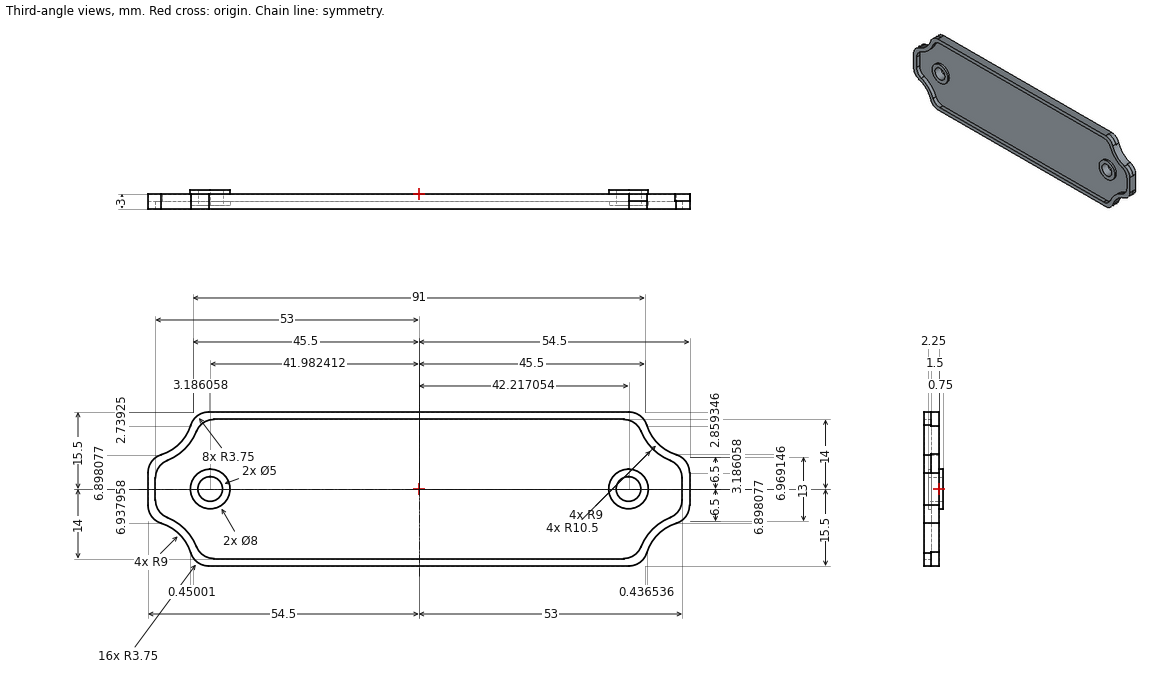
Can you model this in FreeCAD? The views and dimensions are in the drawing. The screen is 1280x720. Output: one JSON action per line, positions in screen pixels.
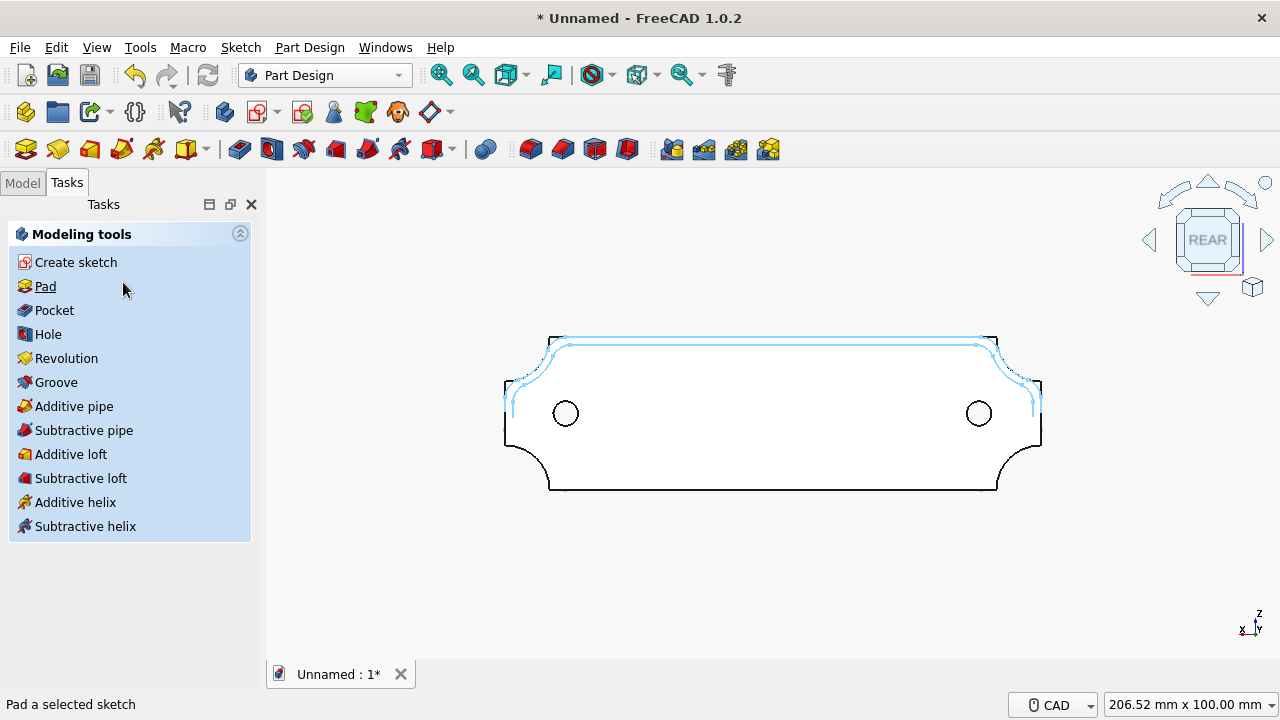
{"action": "left_click", "coordinate": [26, 150]}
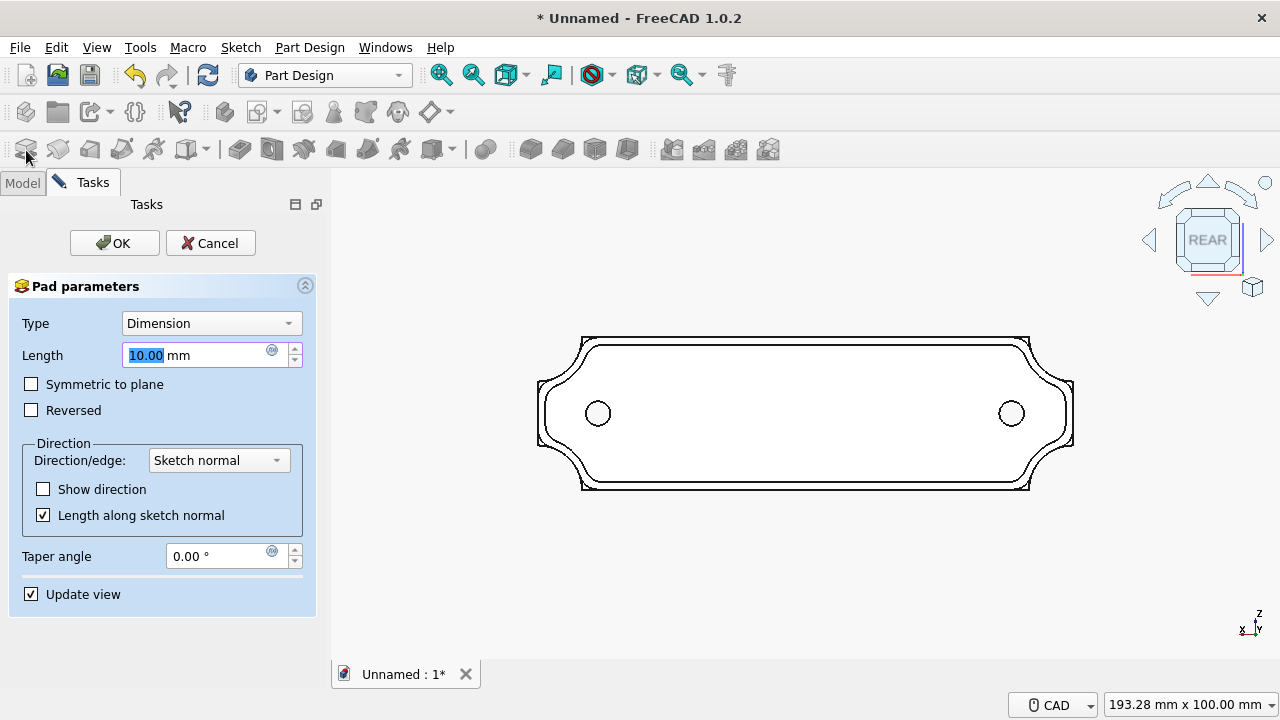
{"action": "type", "text": "3"}
{"action": "key", "text": "Tab"}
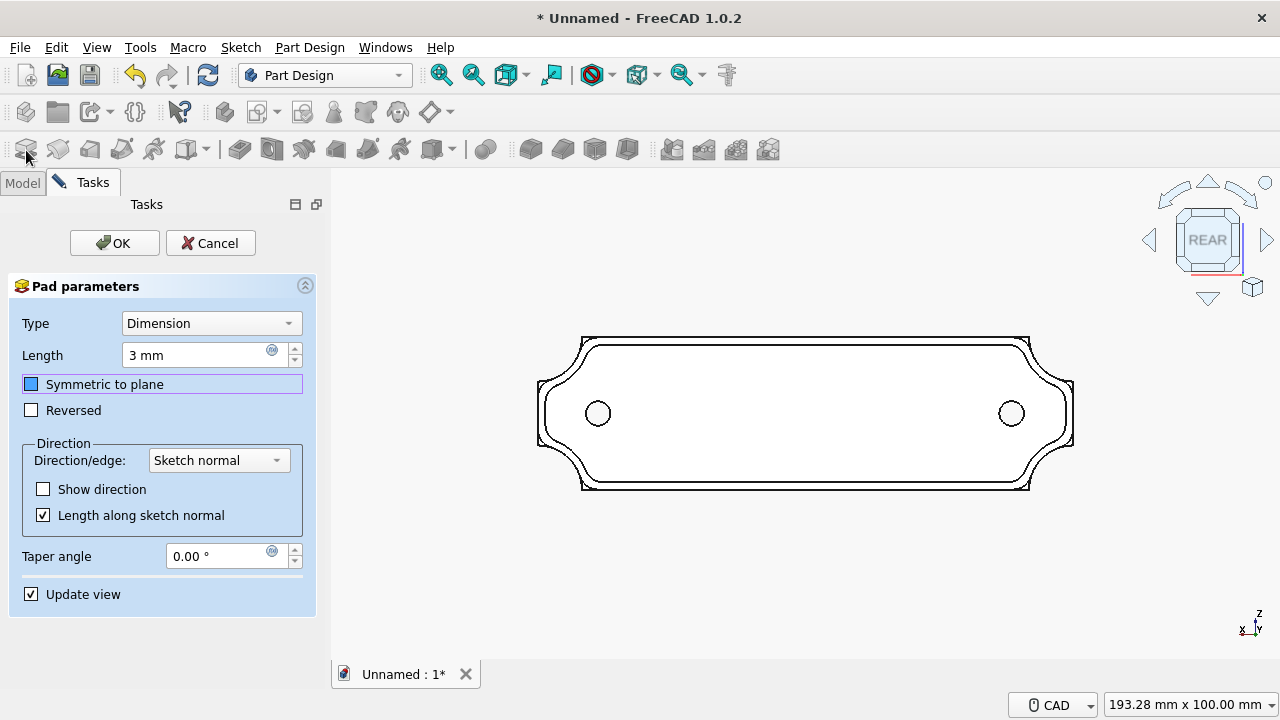
{"action": "left_click", "coordinate": [30, 410]}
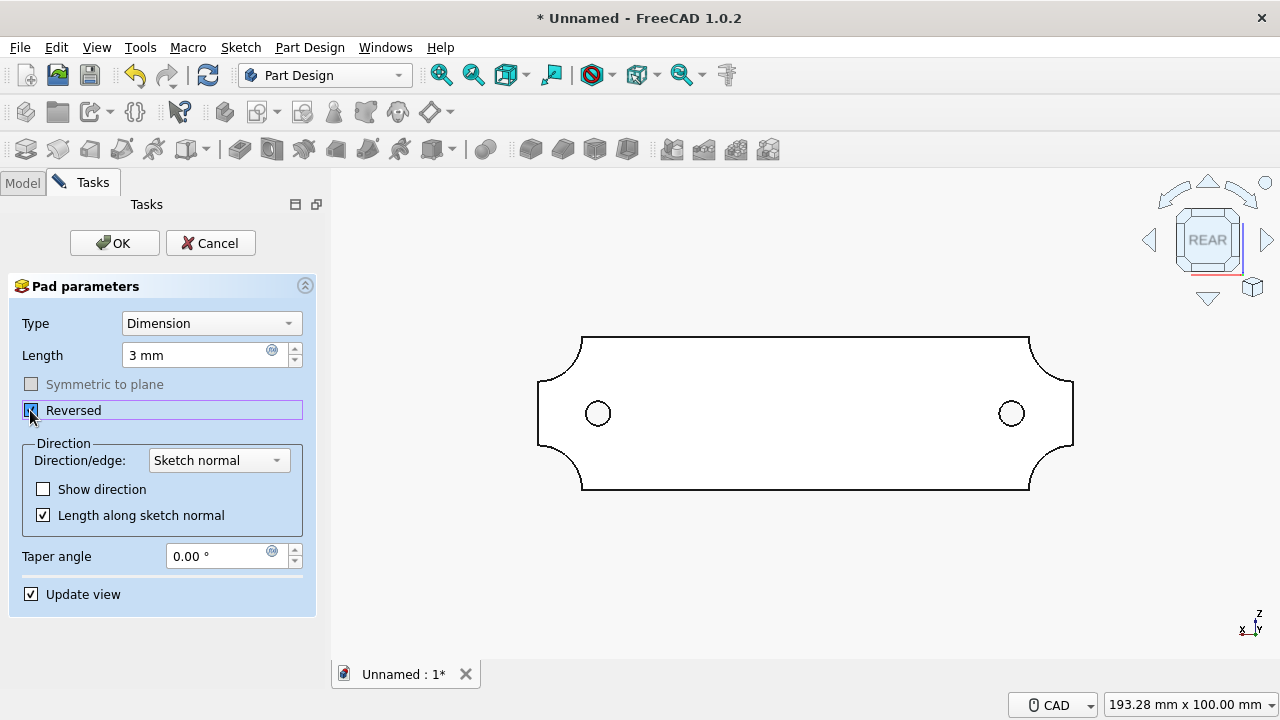
{"action": "left_click", "coordinate": [115, 243]}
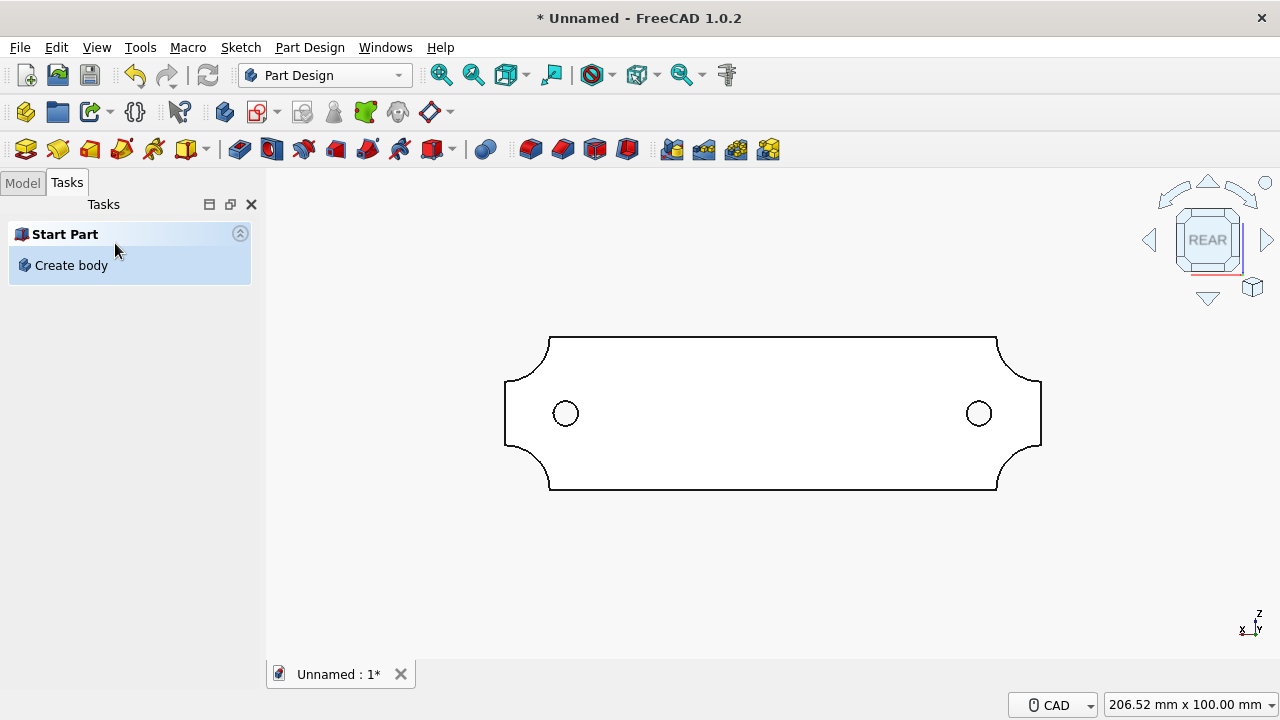
{"action": "left_click", "coordinate": [23, 182]}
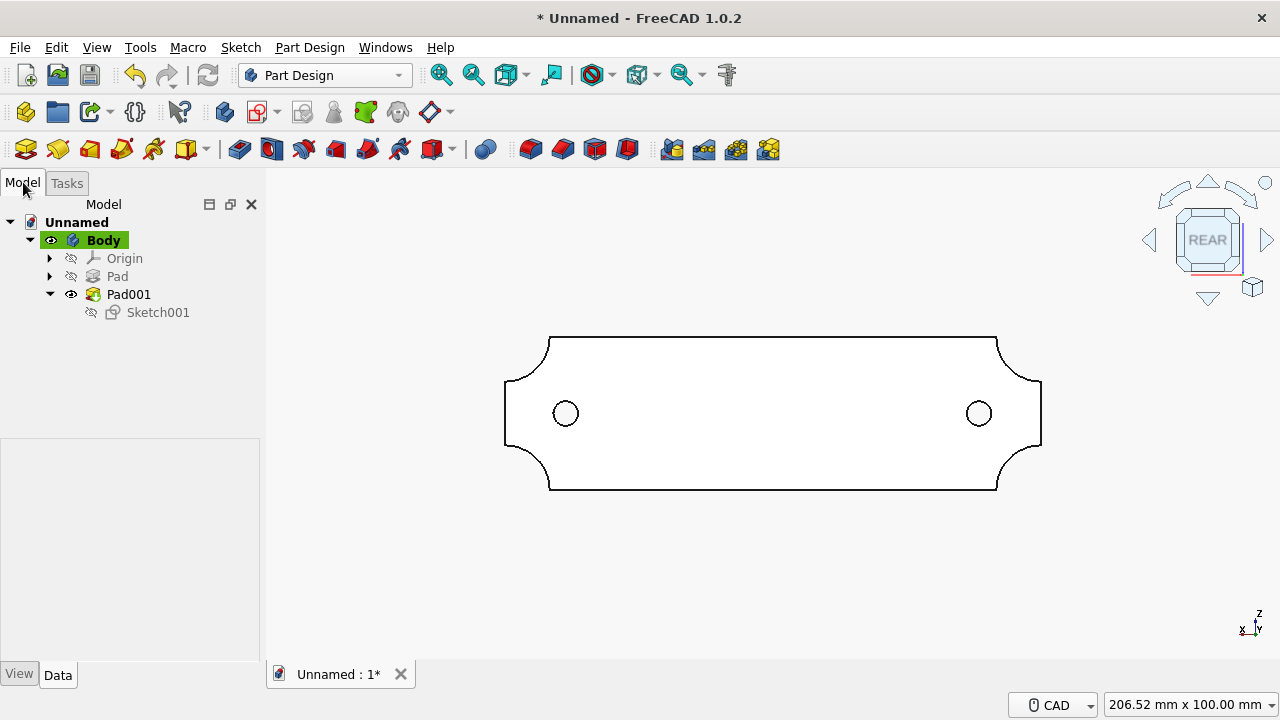
{"action": "left_click", "coordinate": [50, 258]}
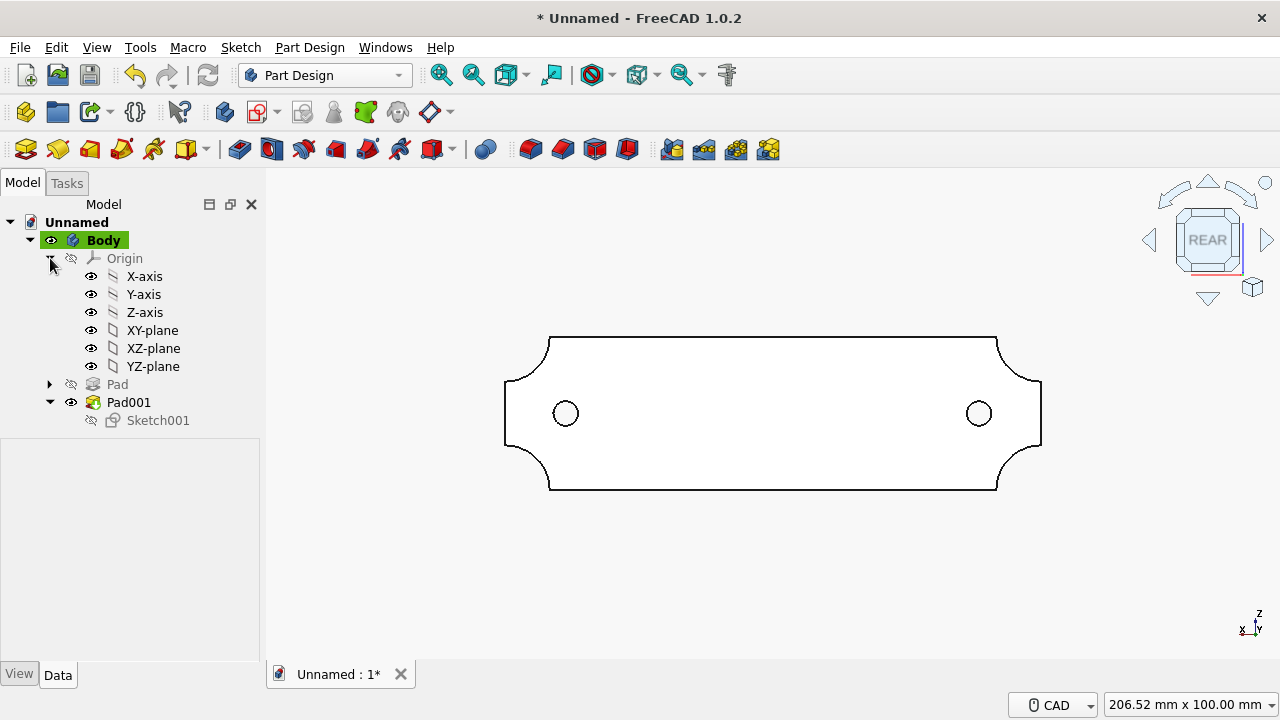
{"action": "left_click", "coordinate": [136, 348]}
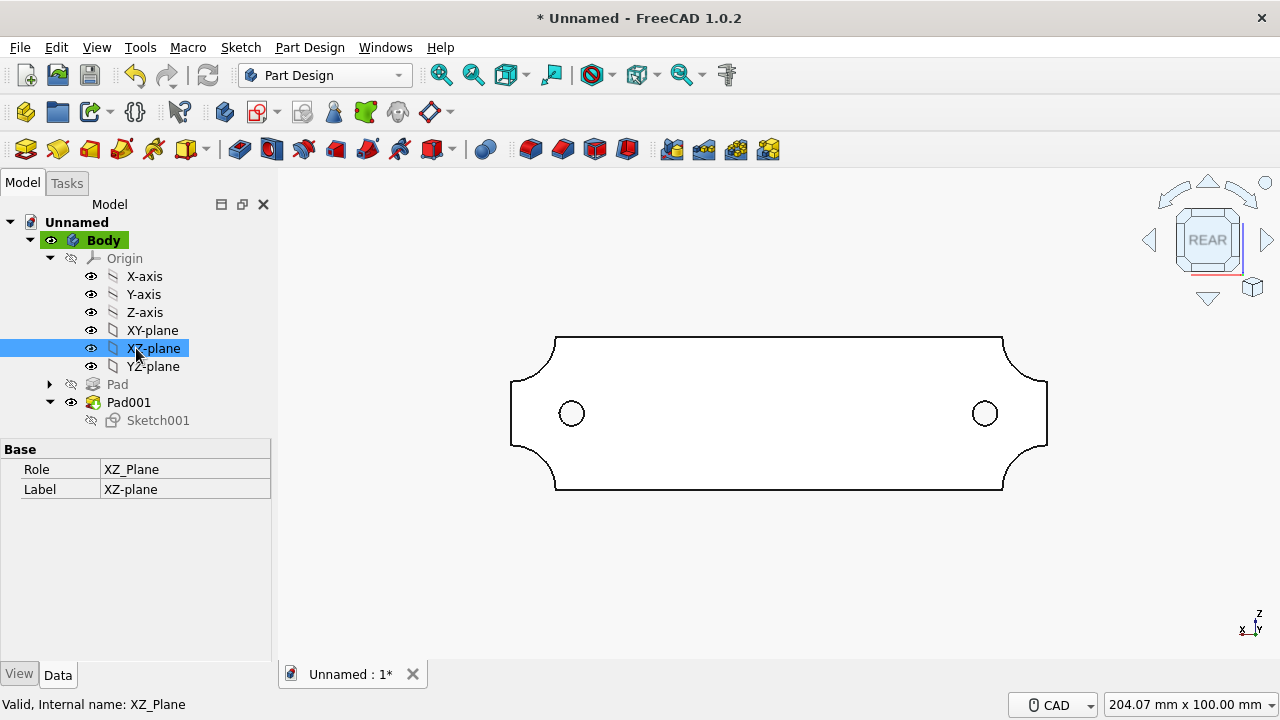
{"action": "left_click", "coordinate": [430, 112]}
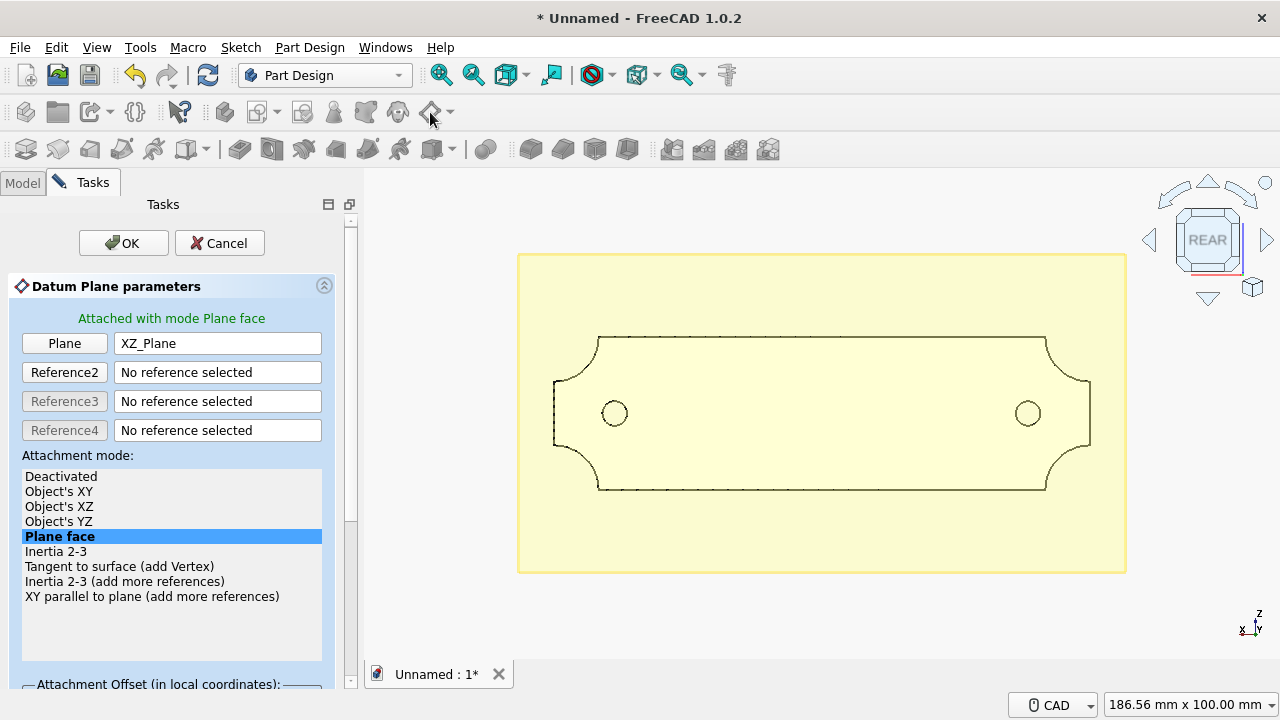
{"action": "scroll", "coordinate": [351, 451], "scroll_direction": "down", "scroll_amount": 3}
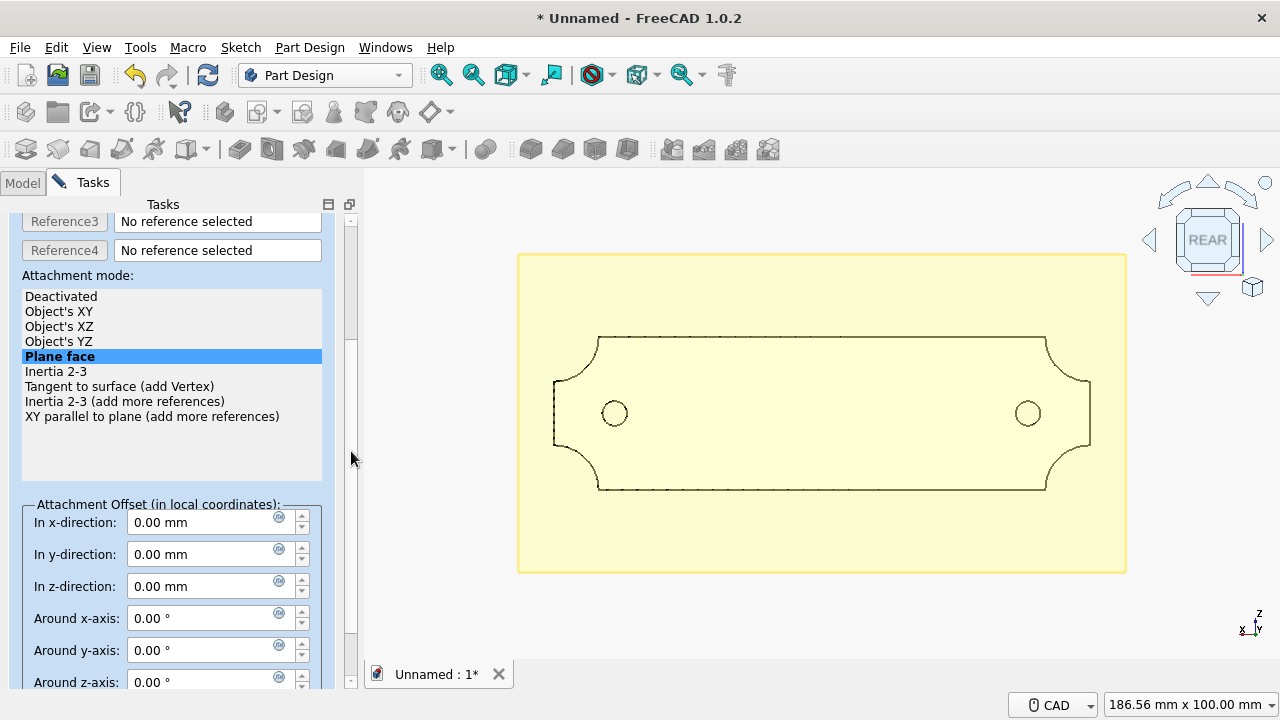
{"action": "triple_click", "coordinate": [210, 586]}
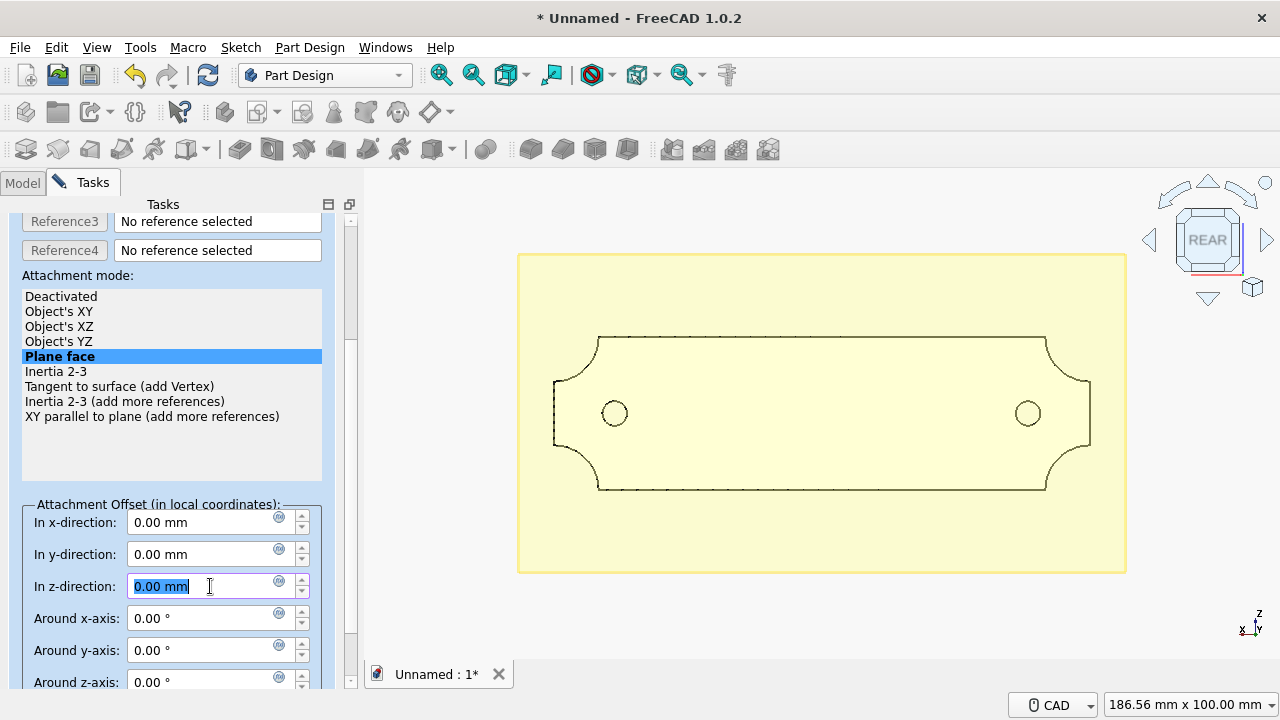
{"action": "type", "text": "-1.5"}
{"action": "key", "text": "Tab"}